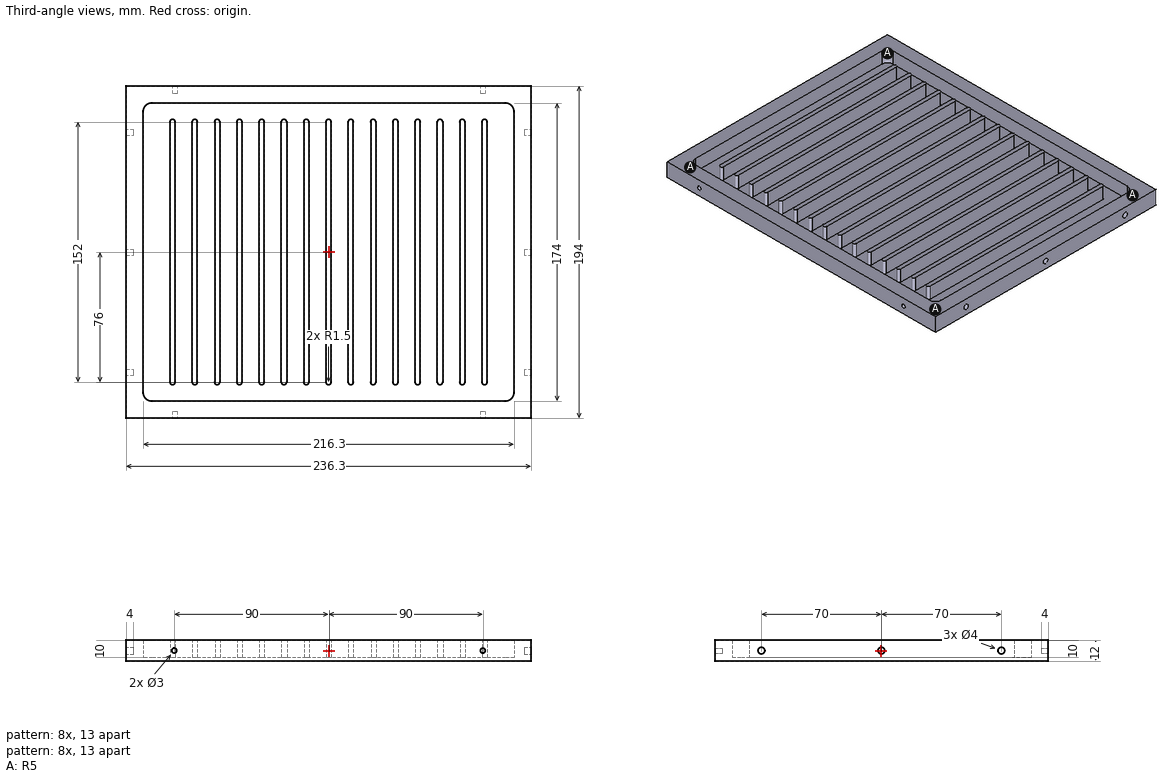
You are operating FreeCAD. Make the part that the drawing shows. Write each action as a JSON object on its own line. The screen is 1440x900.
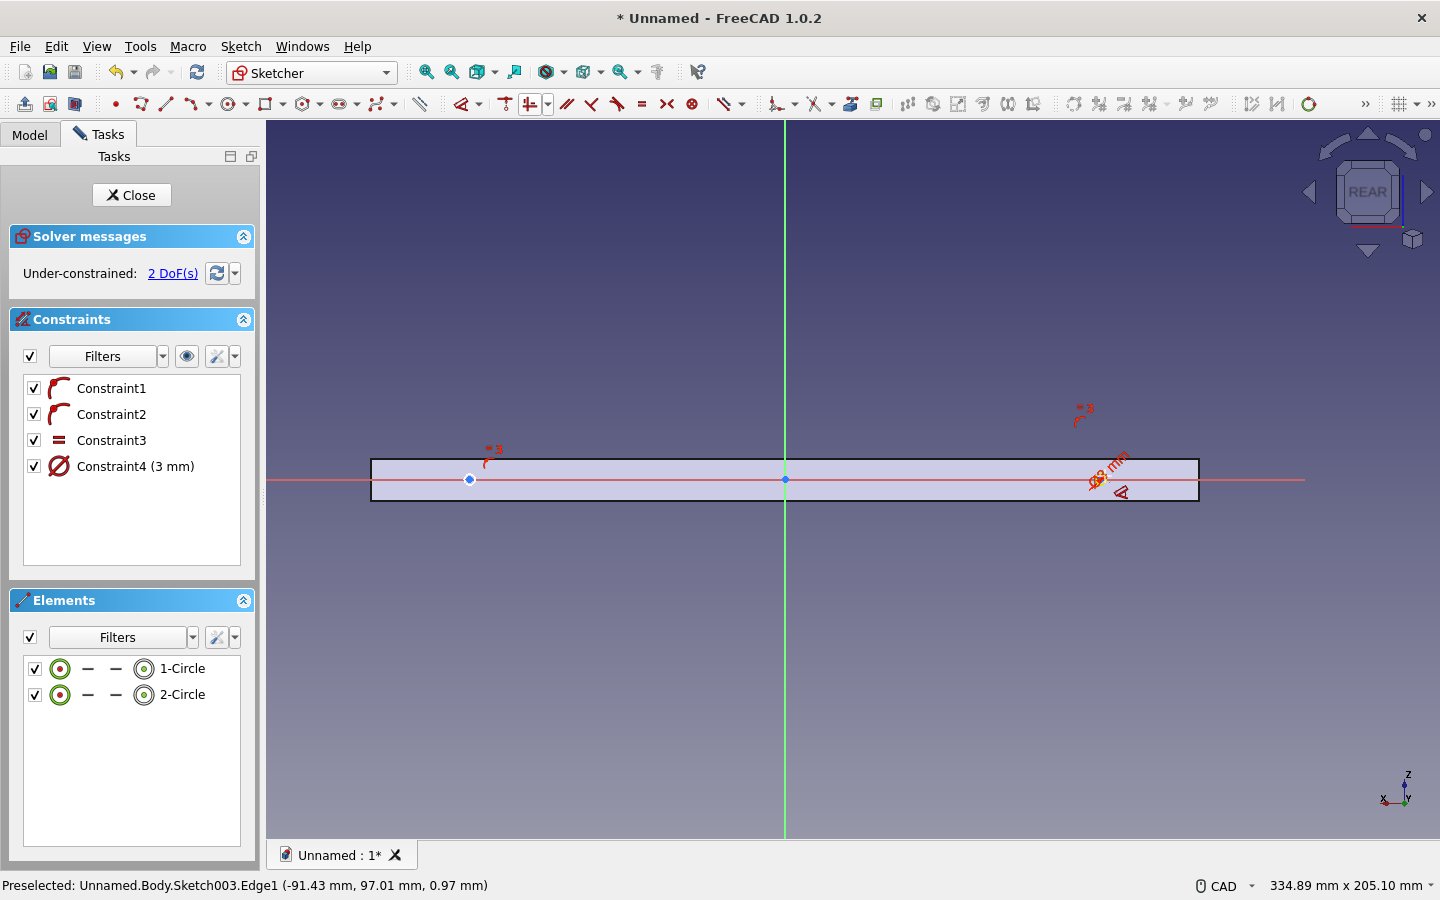
{"action": "left_click", "coordinate": [1101, 480]}
{"action": "left_click", "coordinate": [943, 514]}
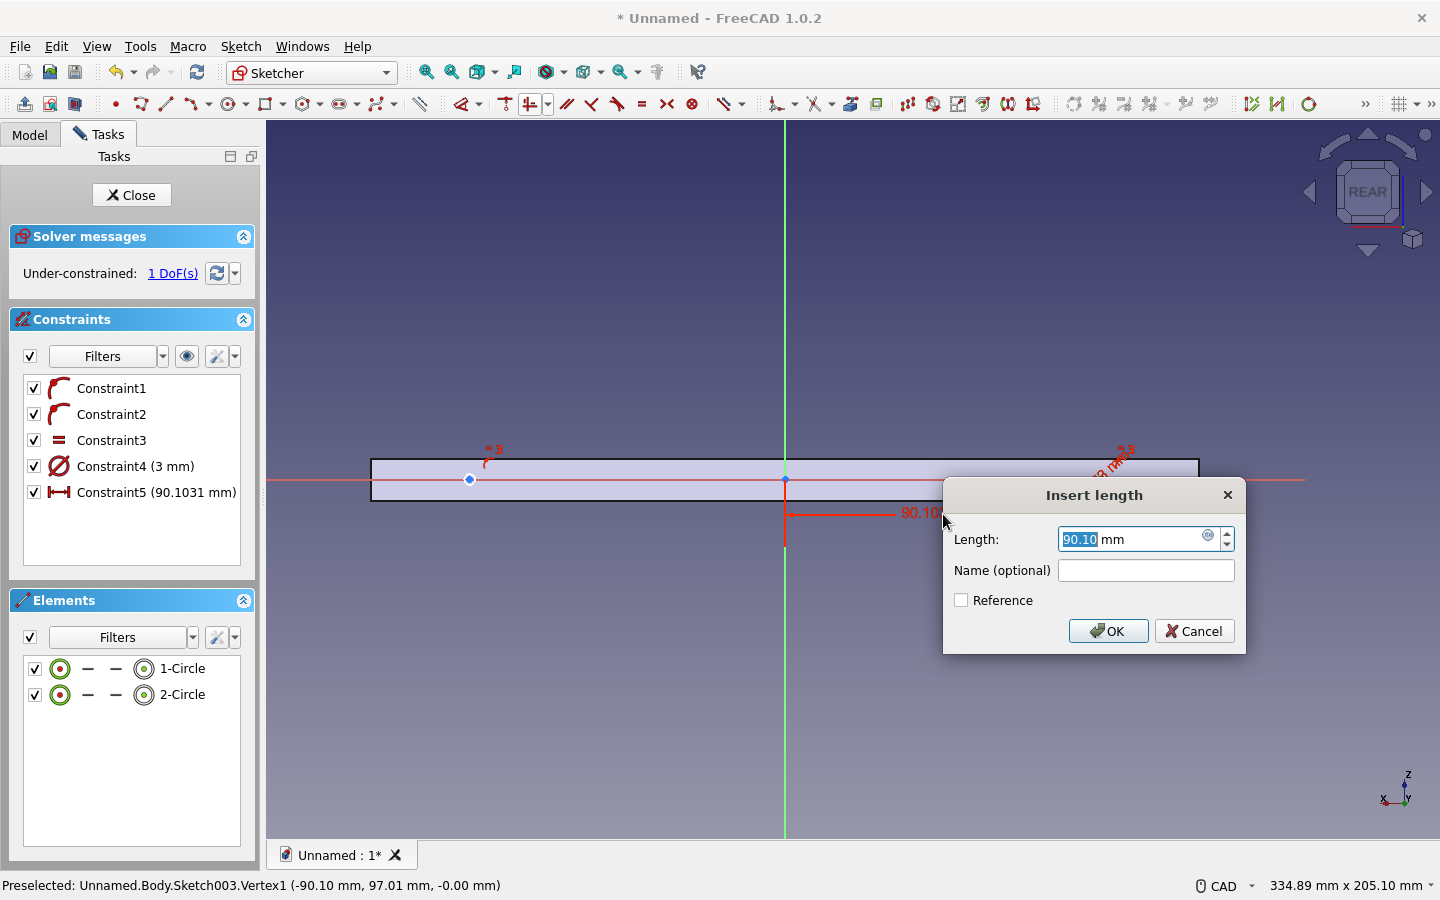
{"action": "type", "text": "90"}
{"action": "key", "text": "Return"}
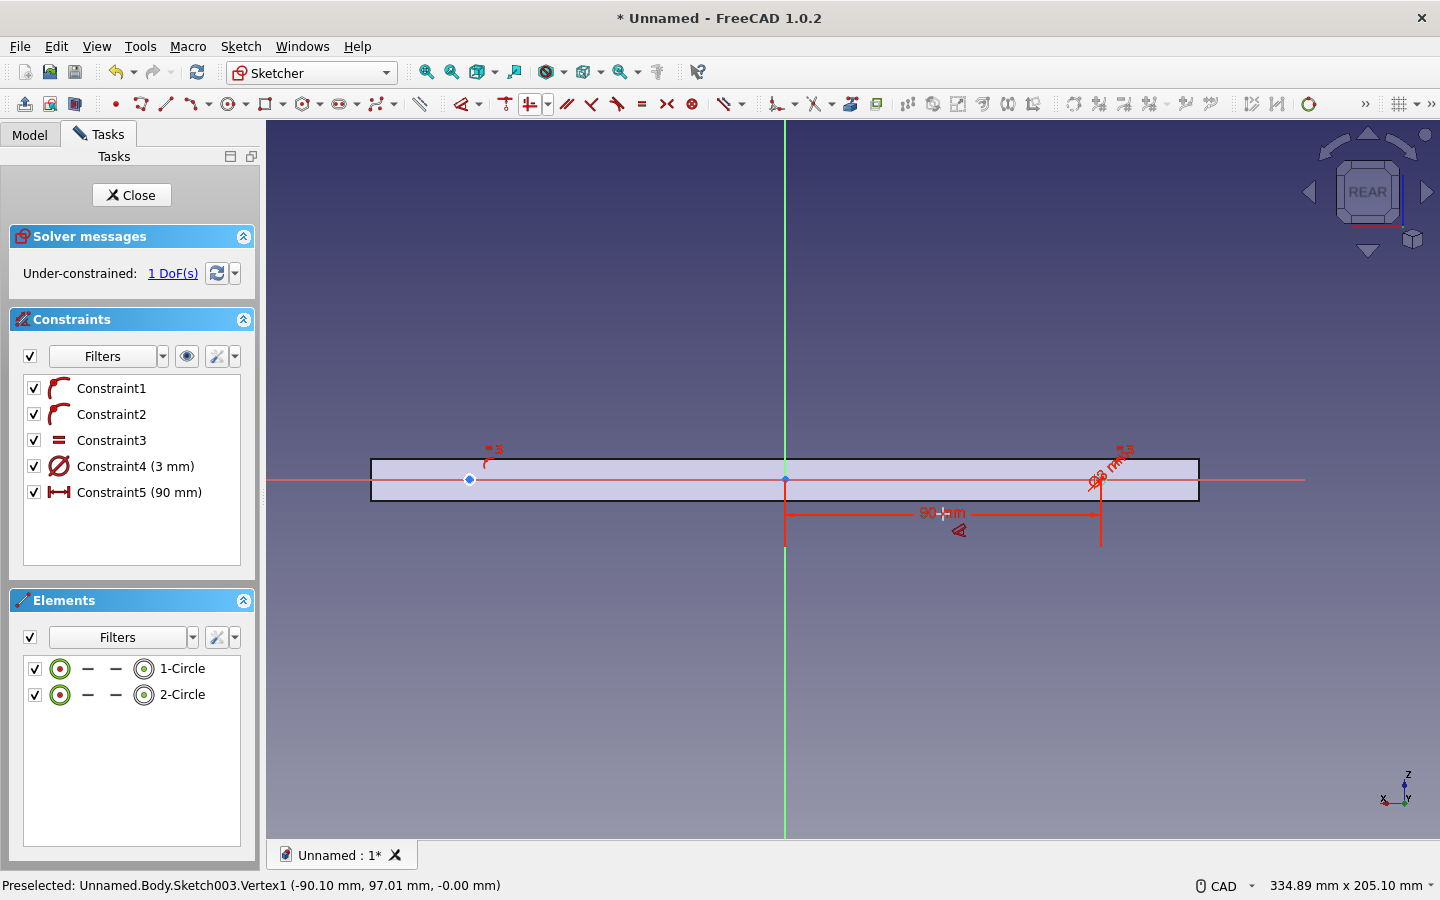
{"action": "left_click", "coordinate": [470, 480]}
{"action": "left_click", "coordinate": [627, 514]}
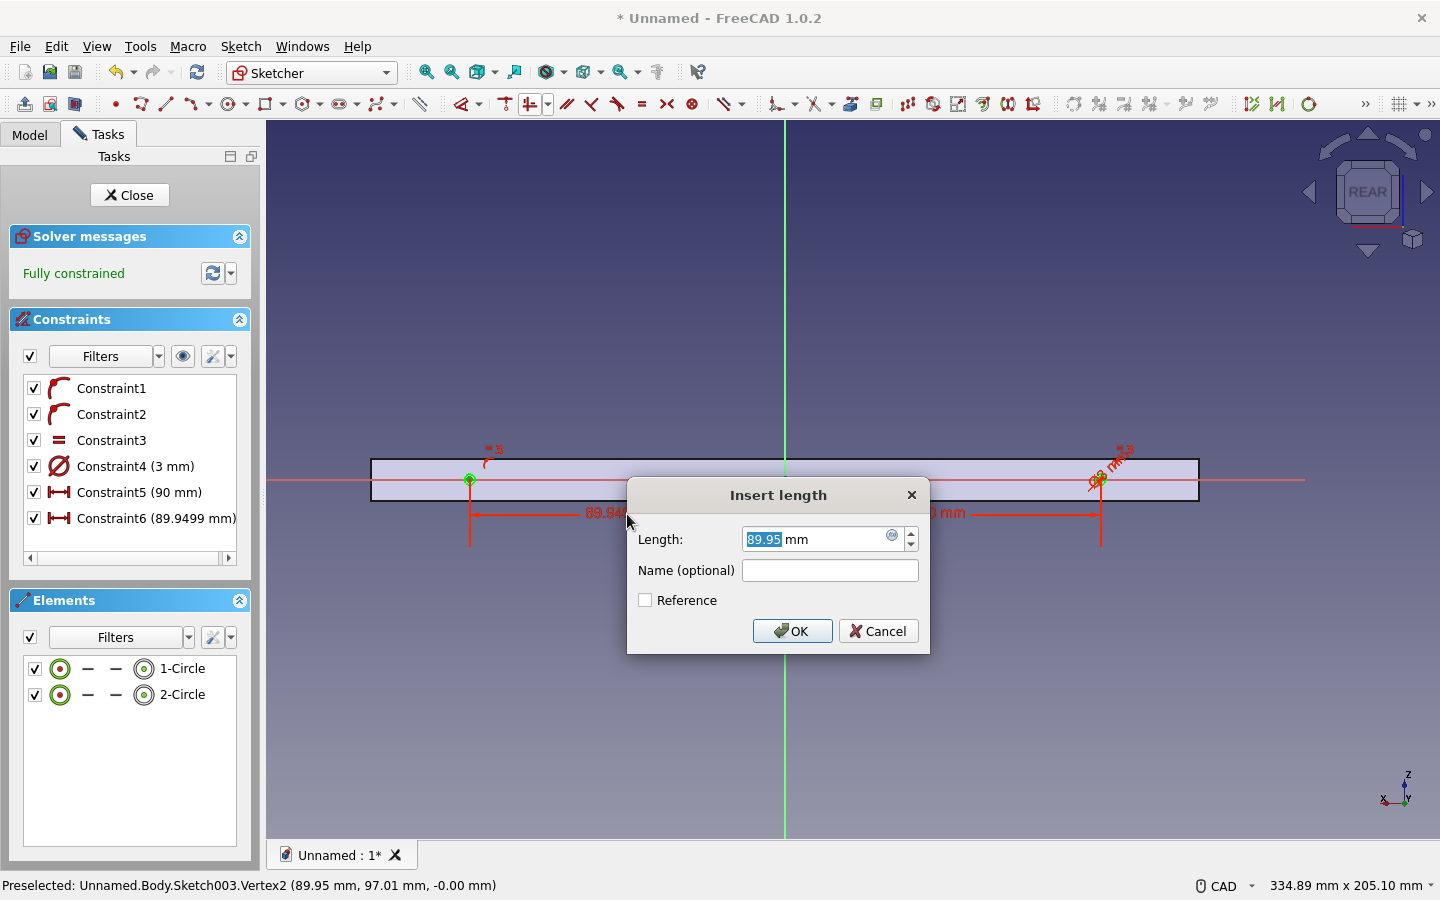
{"action": "type", "text": "90"}
{"action": "key", "text": "Return"}
{"action": "key", "text": "Escape"}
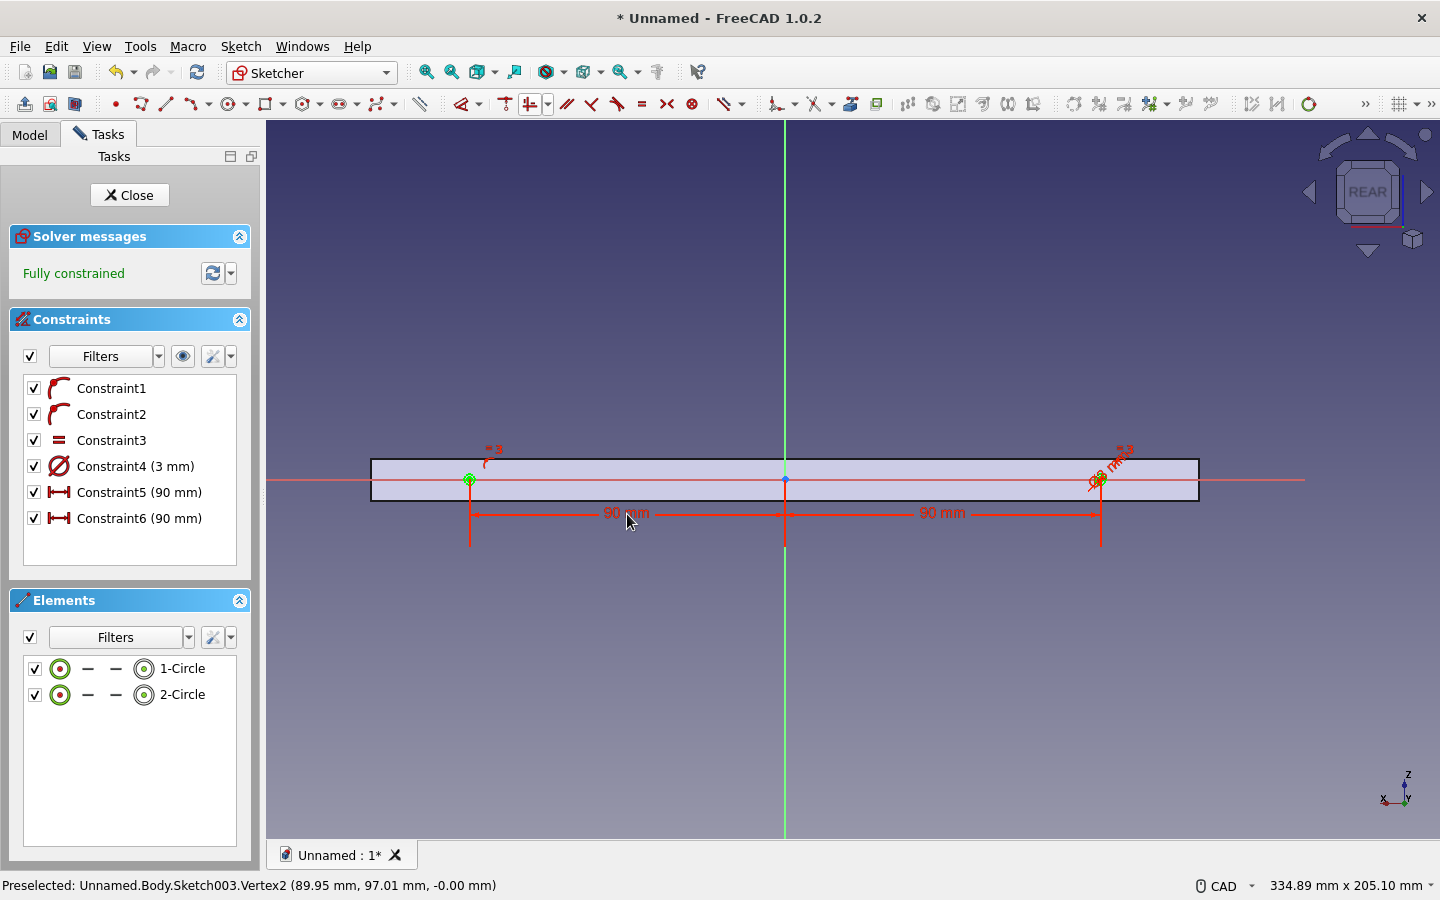
{"action": "left_click", "coordinate": [130, 195]}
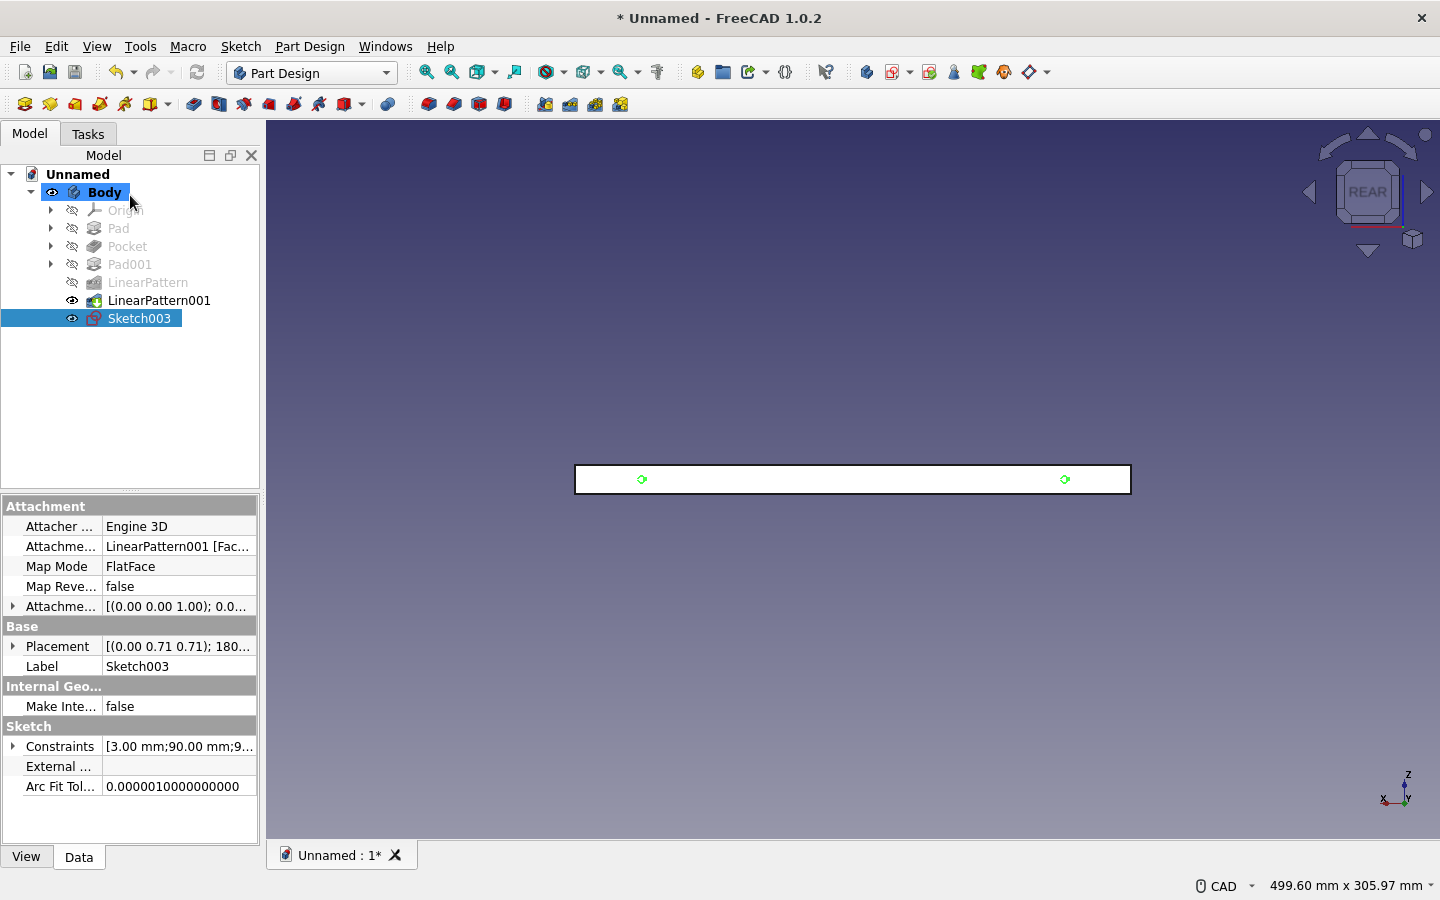
{"action": "left_click", "coordinate": [194, 104]}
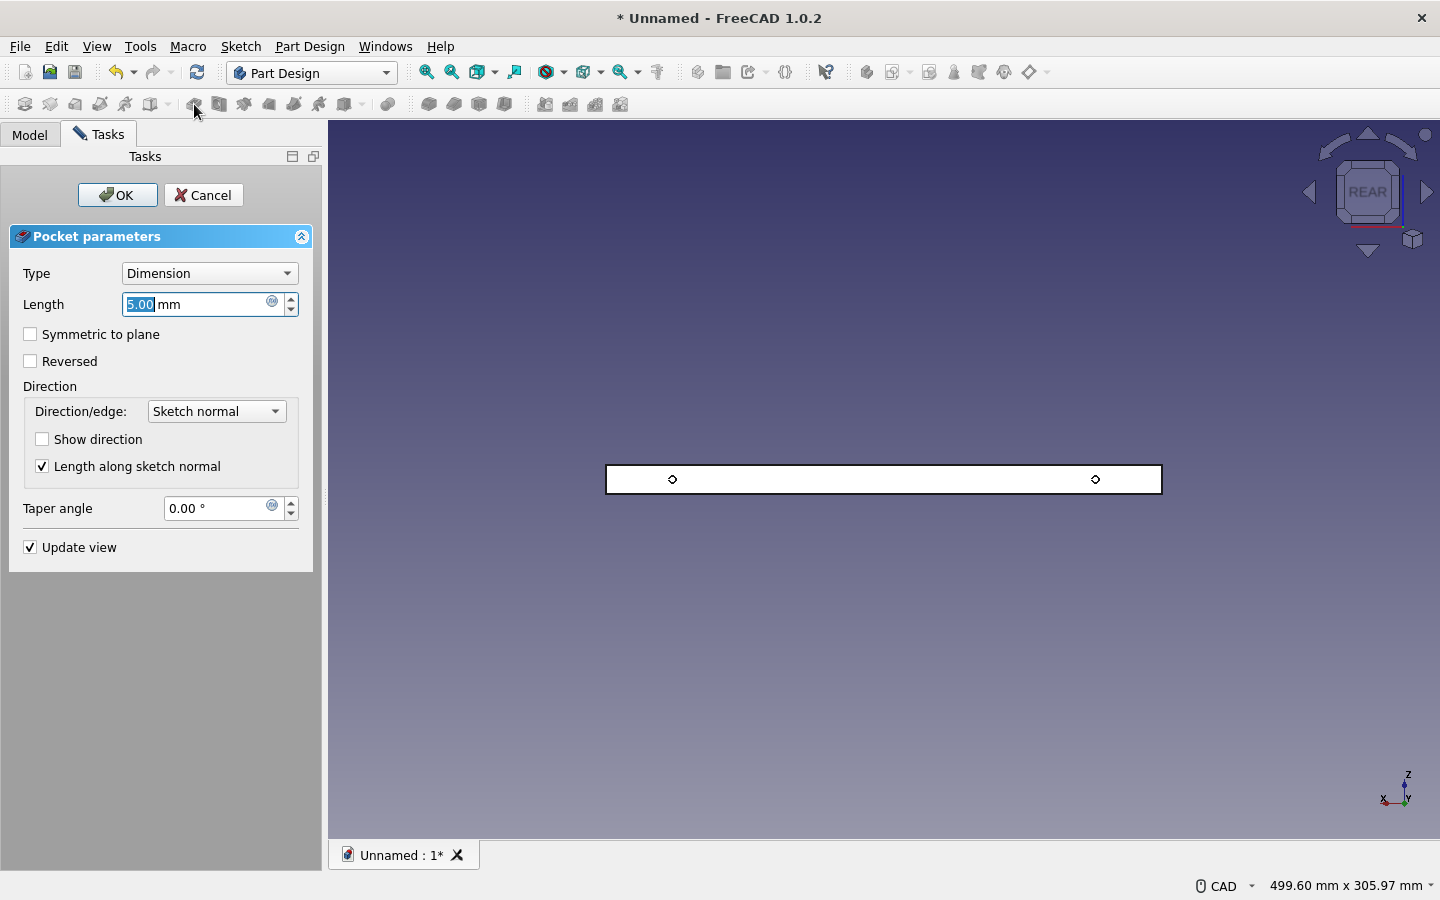
{"action": "type", "text": "4"}
{"action": "key", "text": "Tab"}